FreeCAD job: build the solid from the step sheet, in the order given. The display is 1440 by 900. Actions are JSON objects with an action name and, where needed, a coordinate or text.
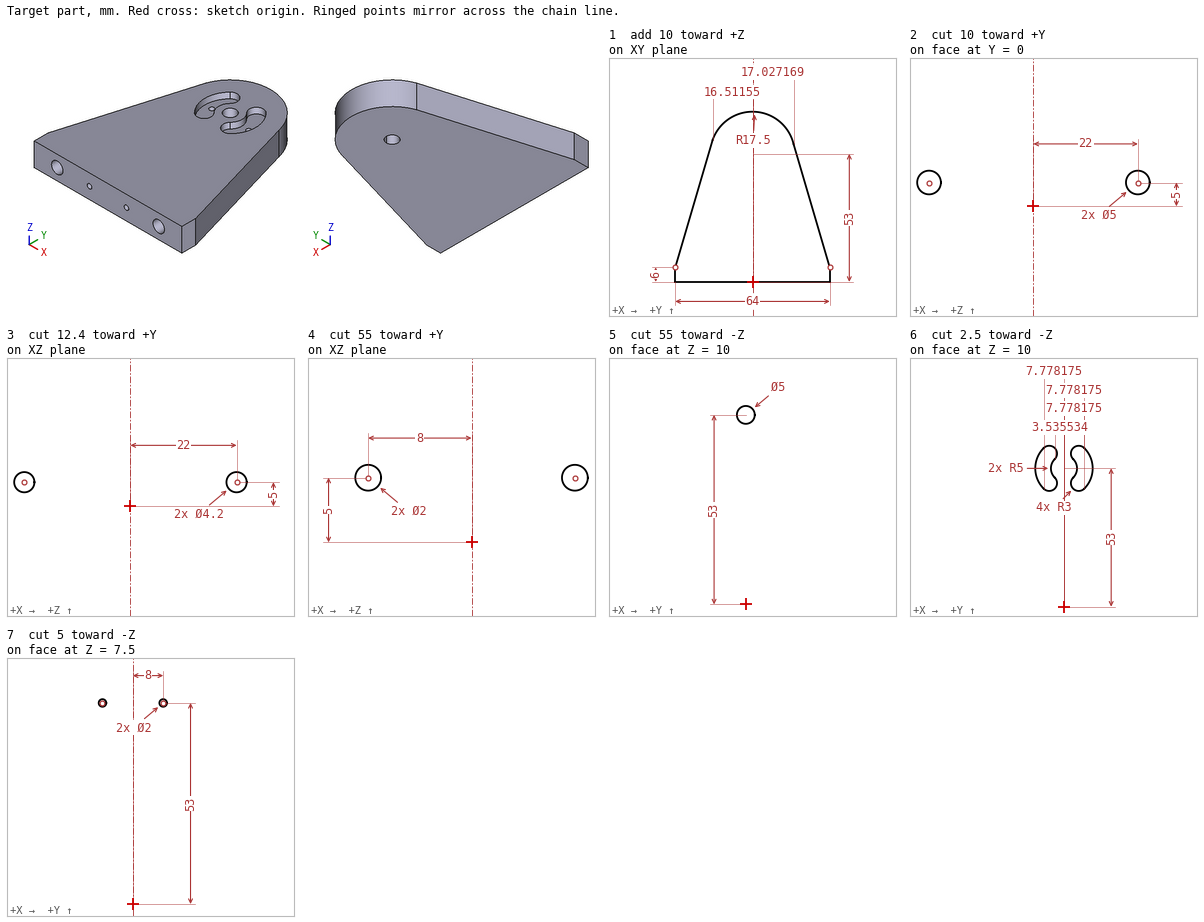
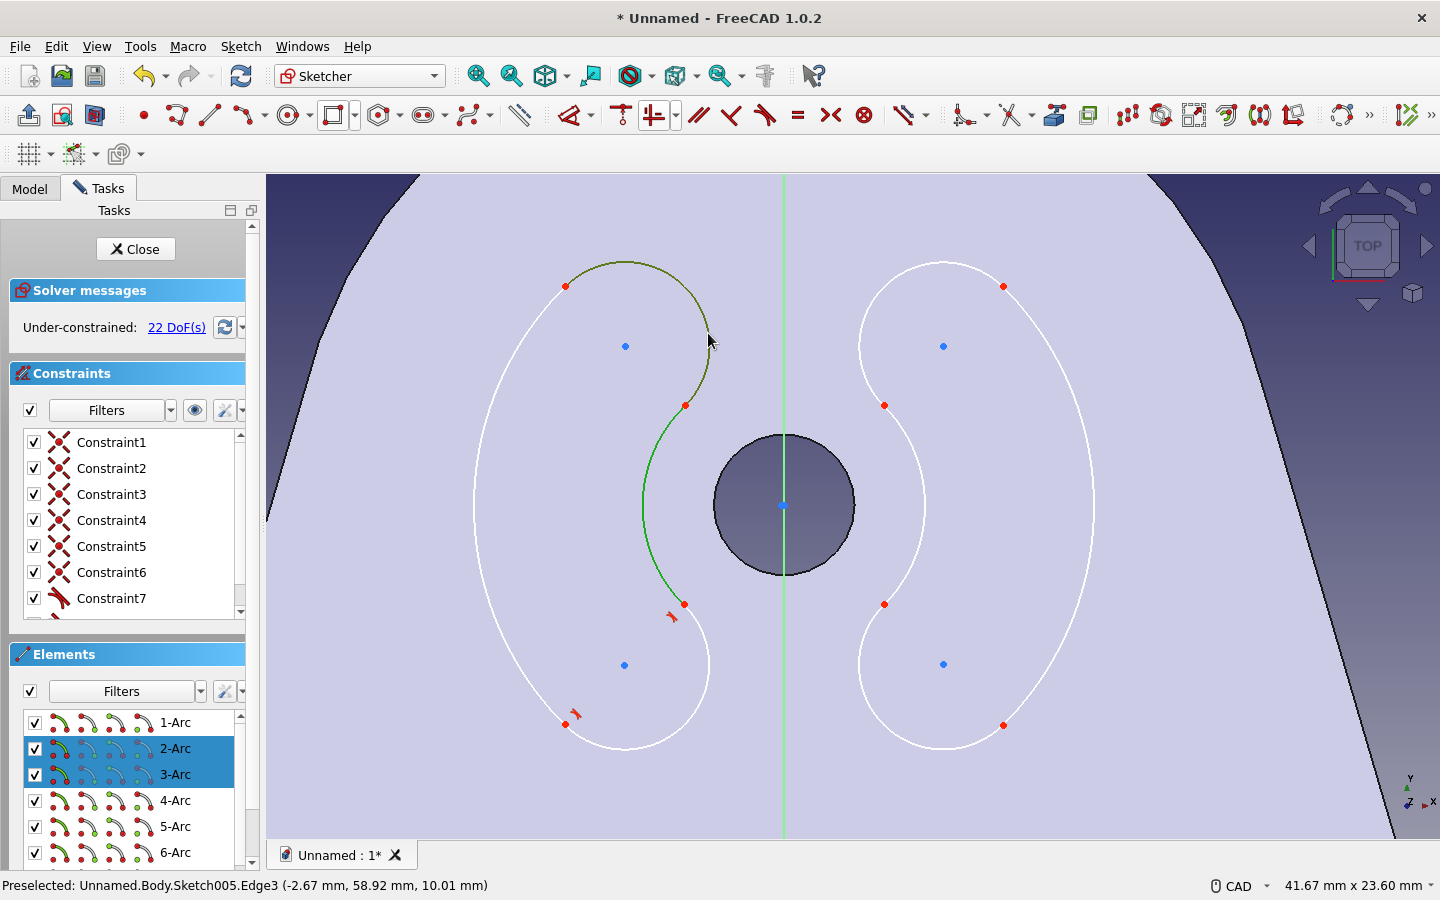
{"action": "left_click", "coordinate": [765, 116]}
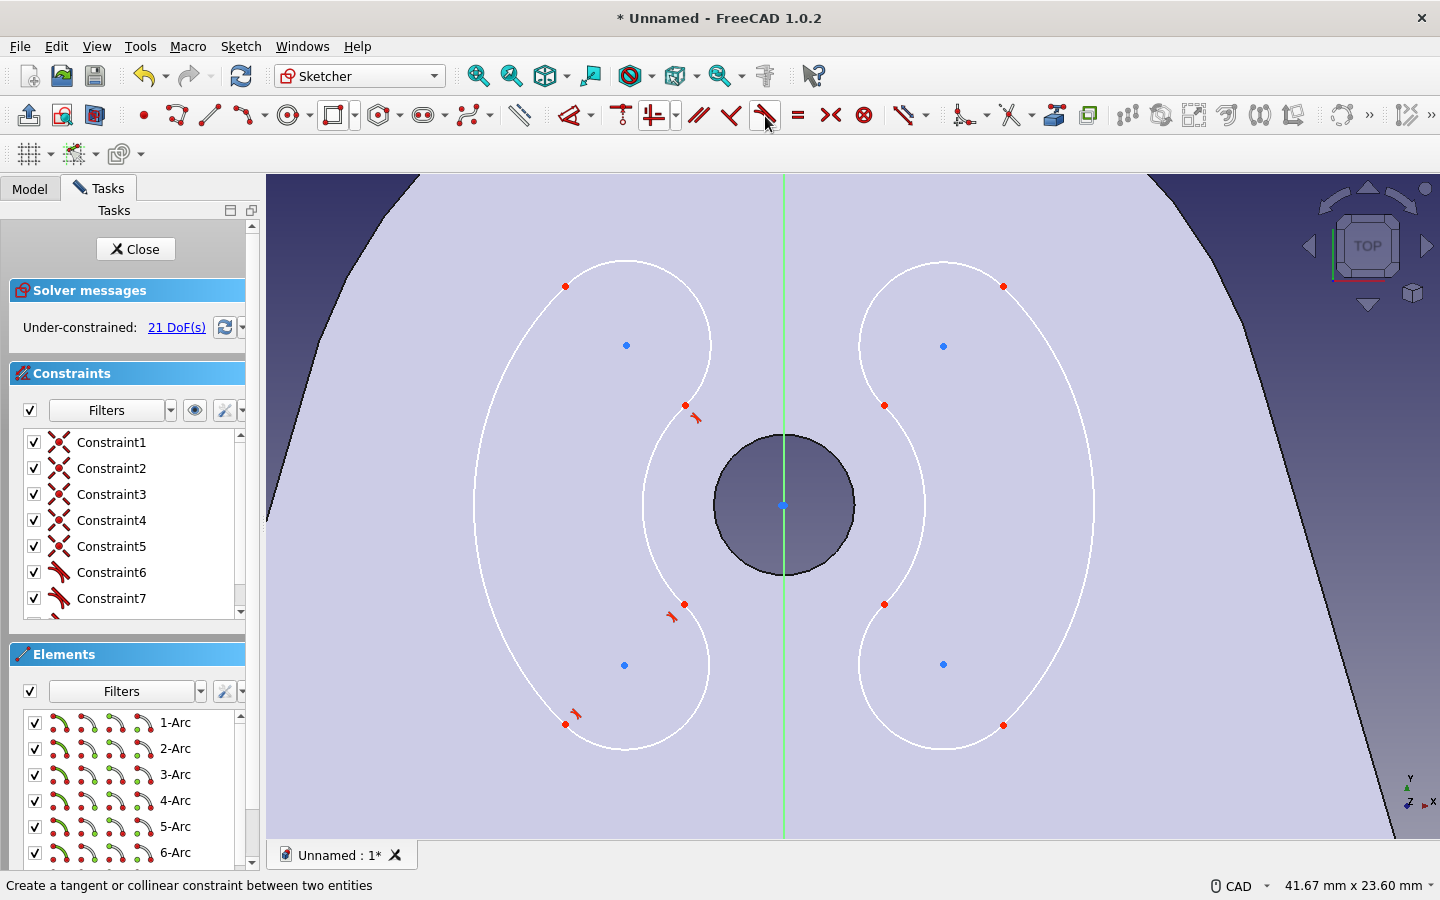
{"action": "left_click", "coordinate": [710, 332]}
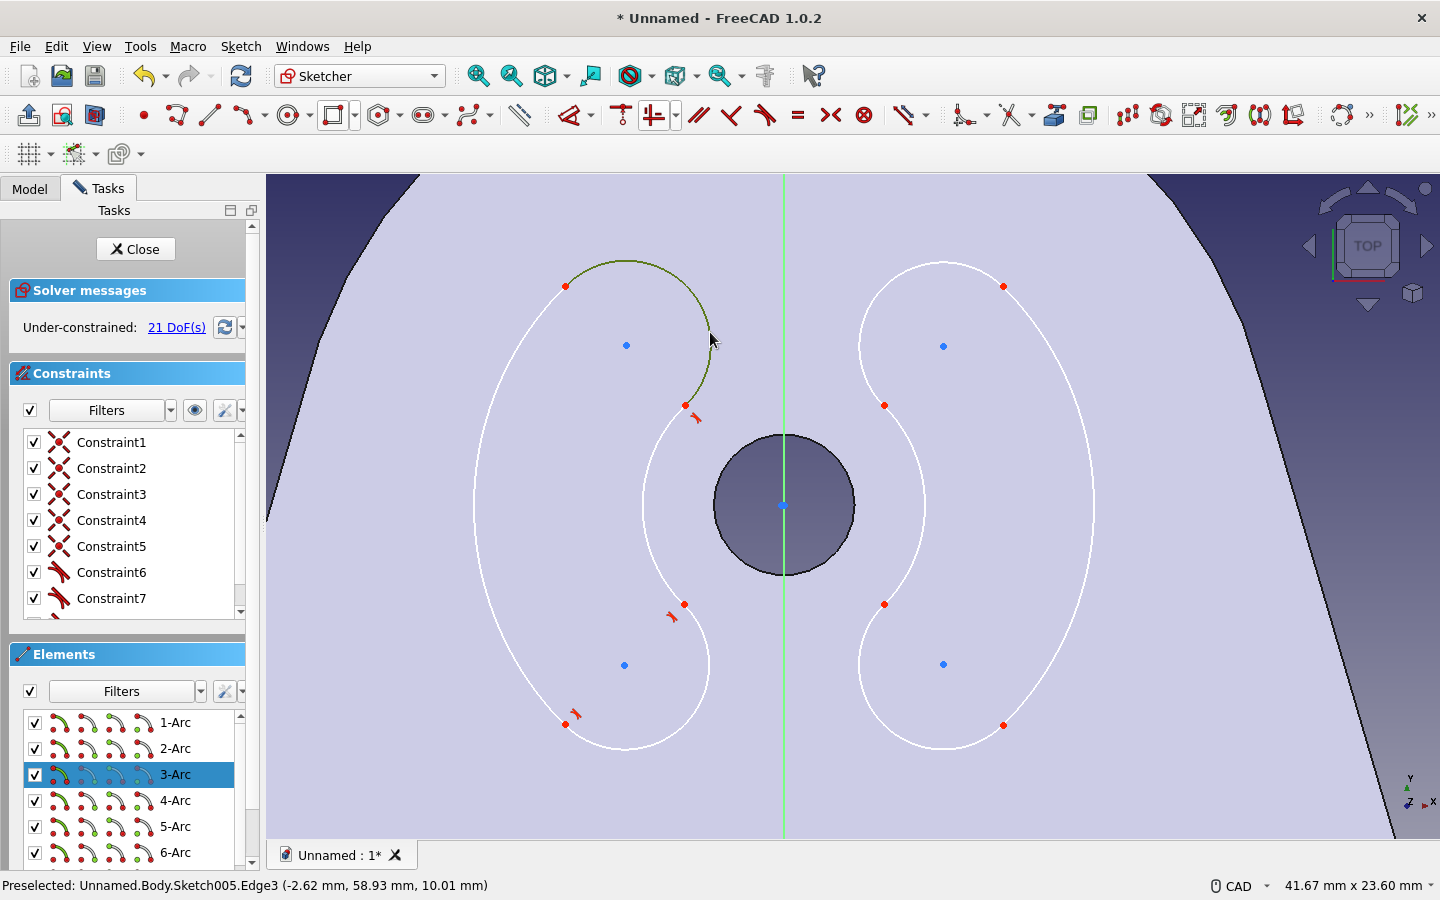
{"action": "left_click", "coordinate": [489, 410]}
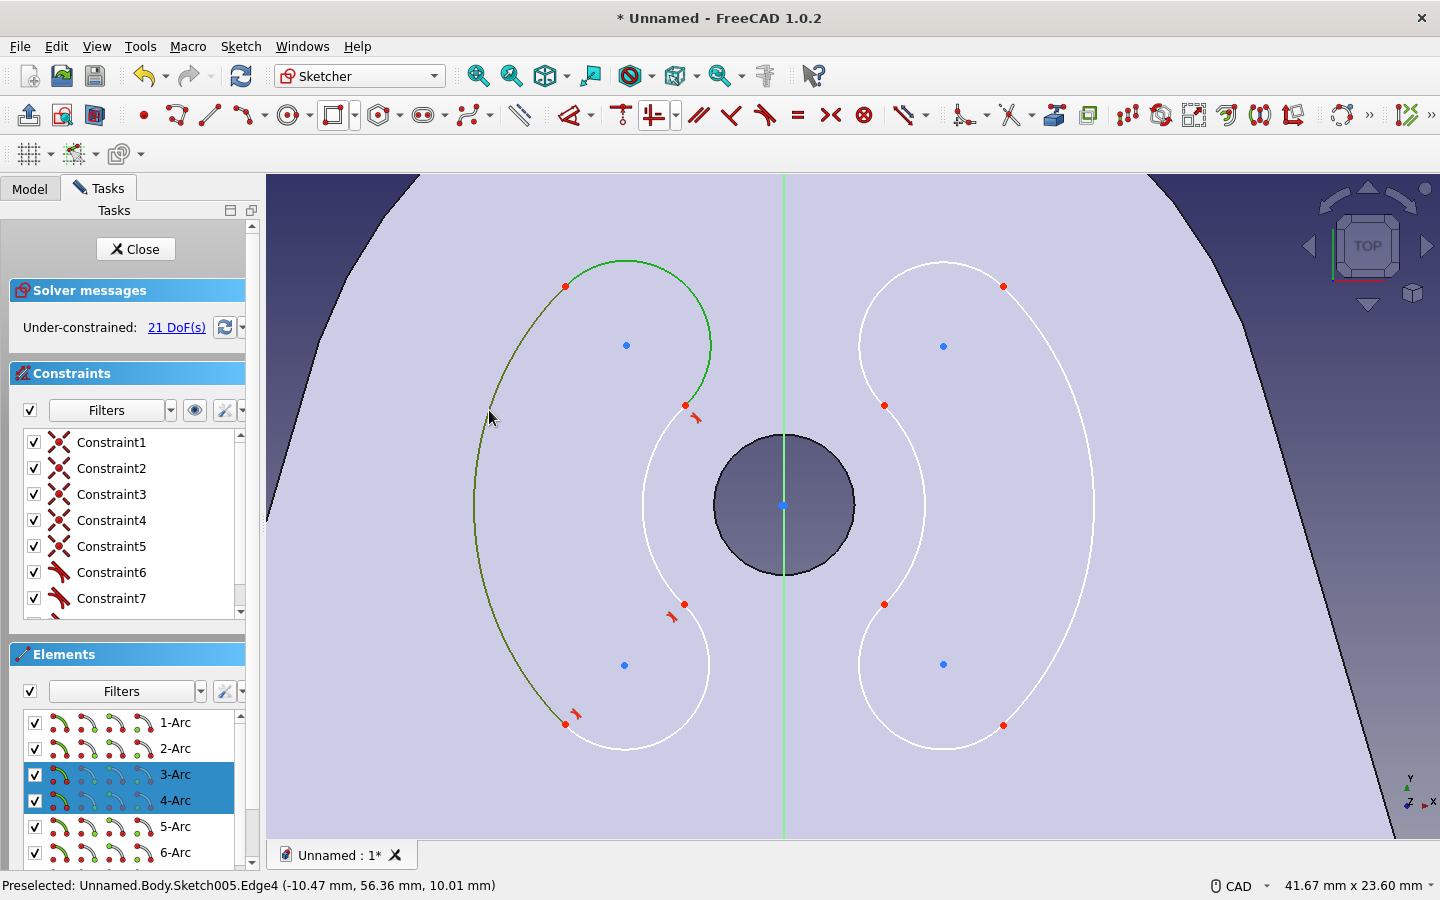
{"action": "key", "text": "t"}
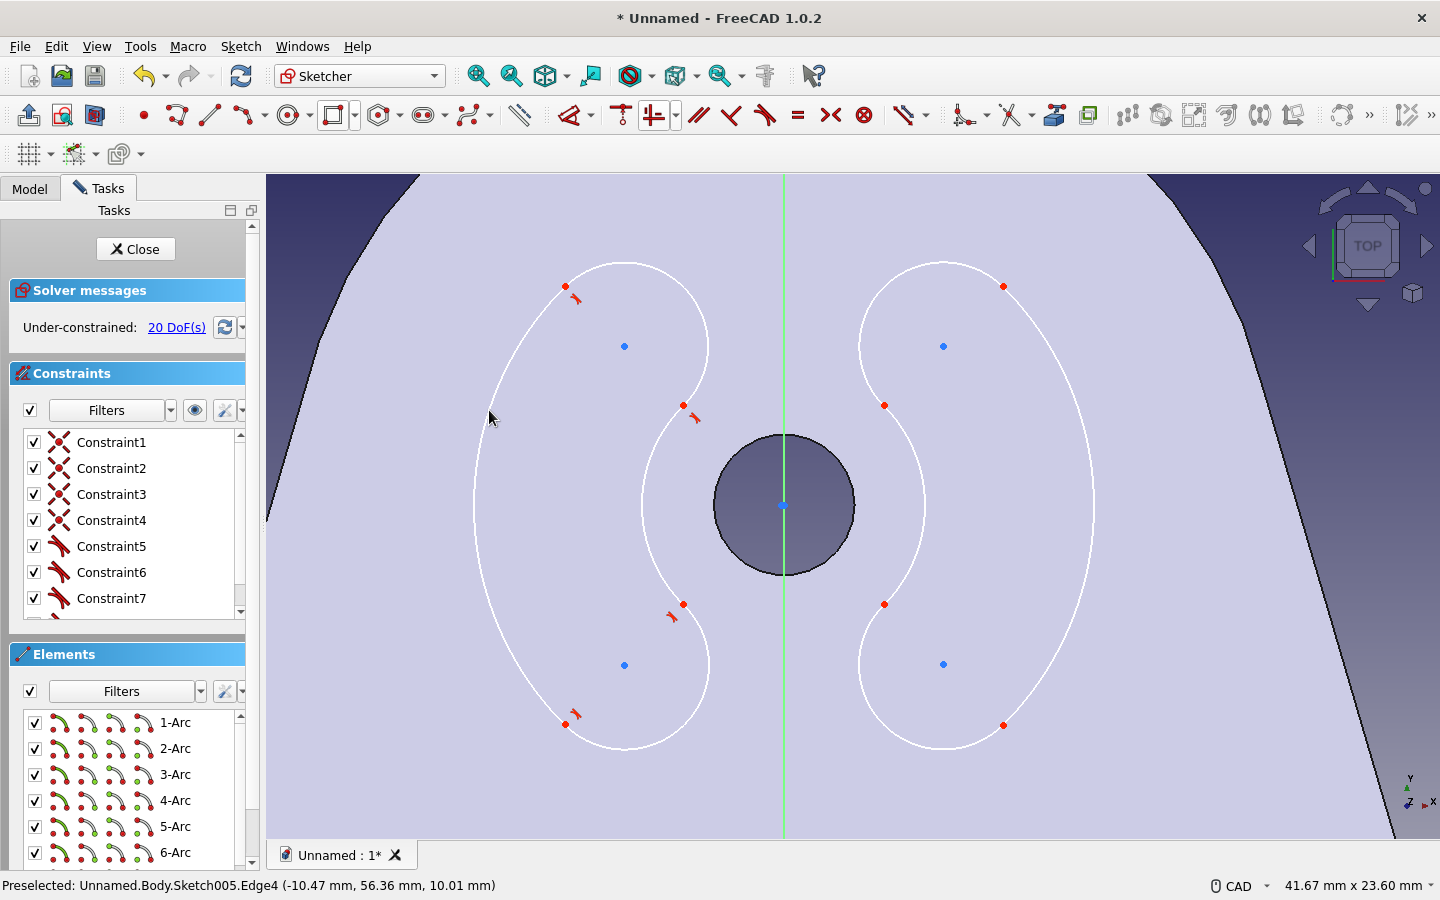
{"action": "left_click", "coordinate": [1079, 602]}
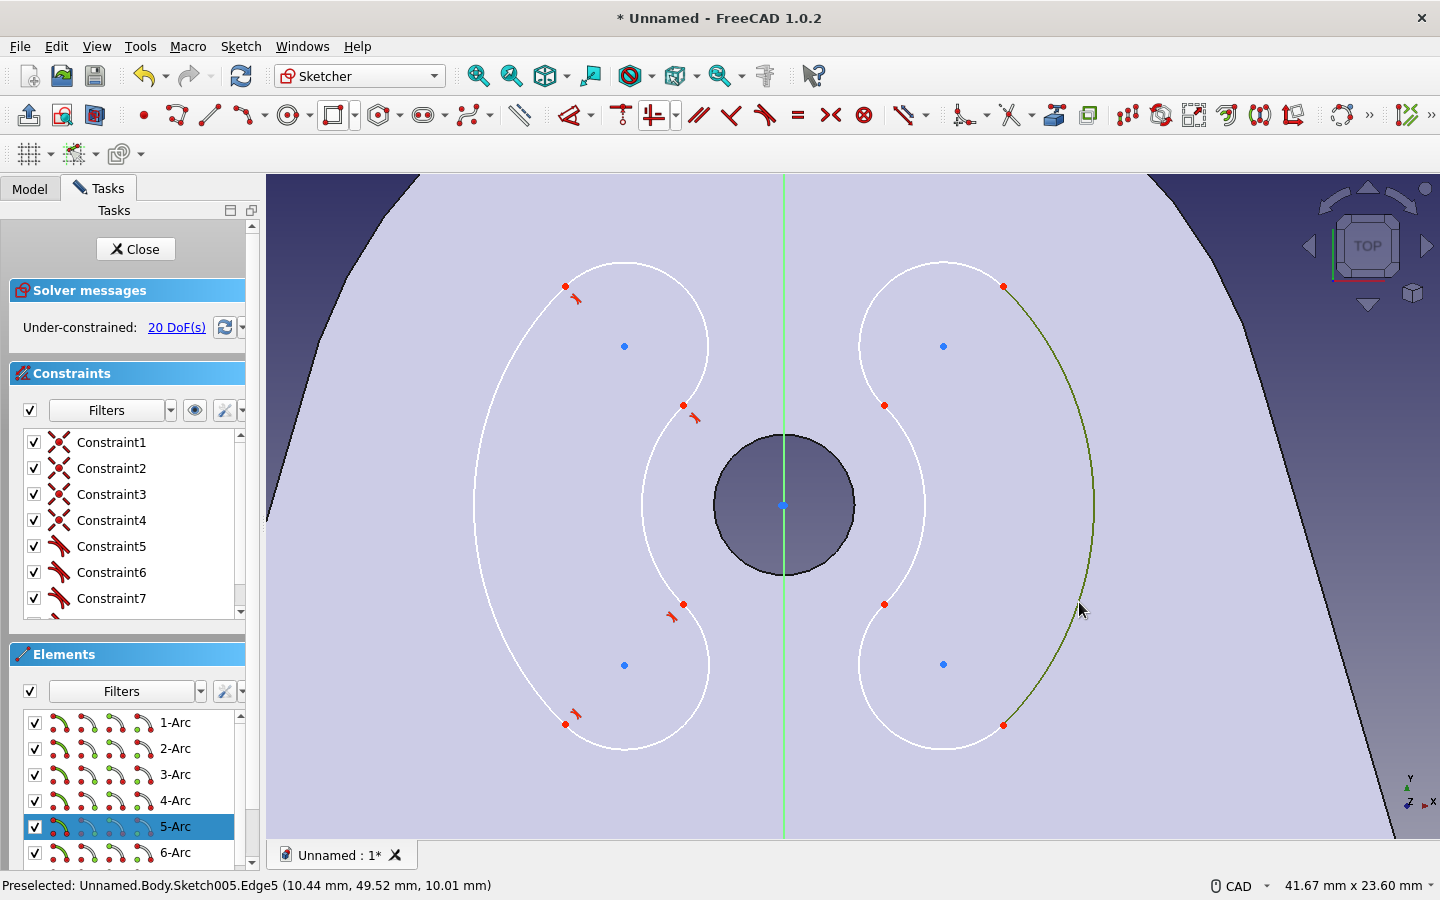
{"action": "left_click", "coordinate": [930, 263]}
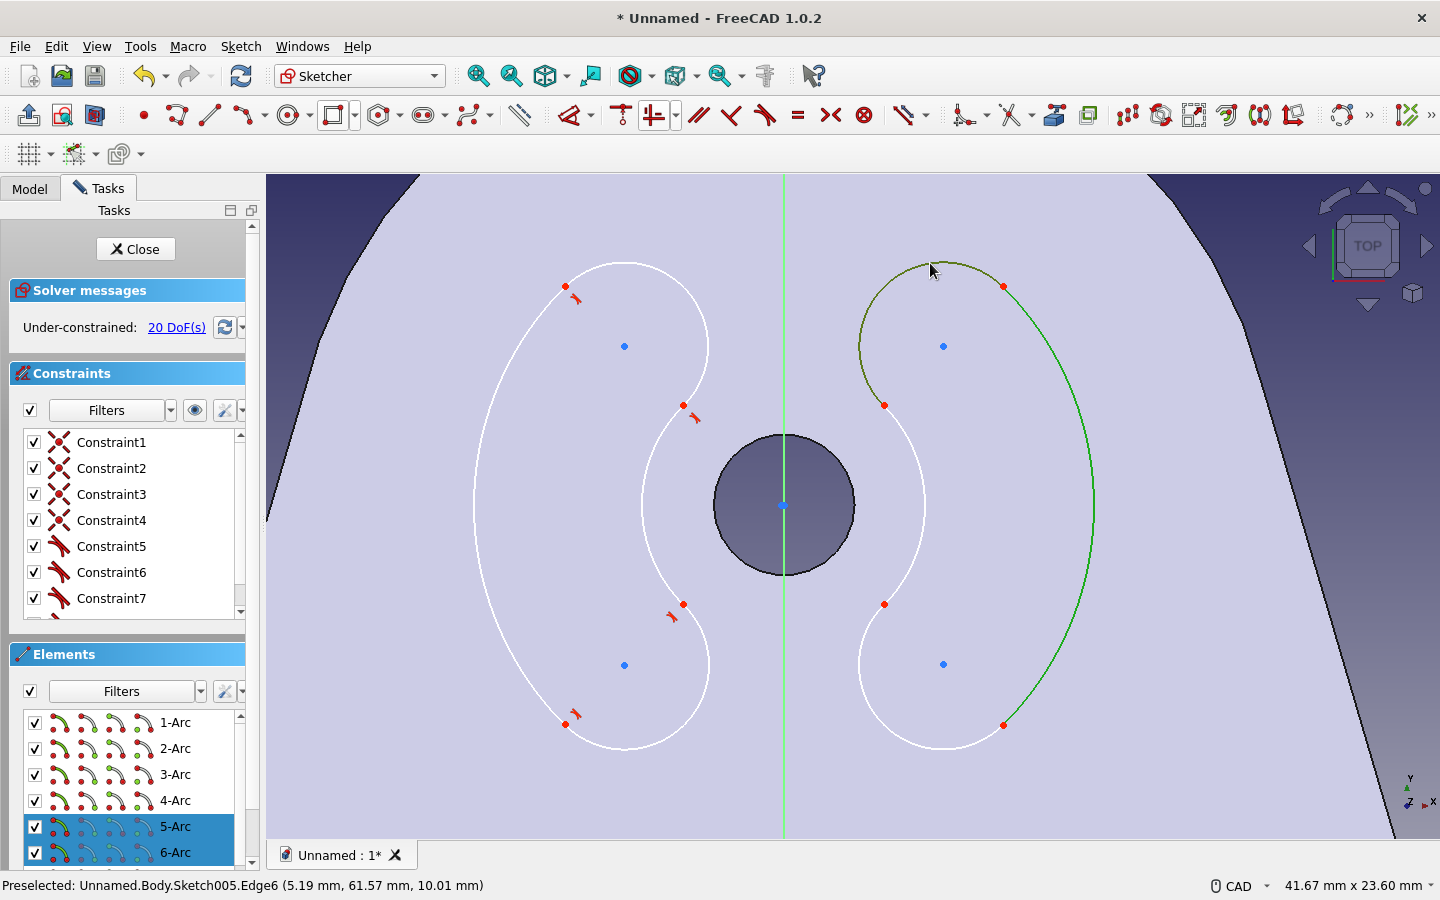
{"action": "left_click", "coordinate": [765, 116]}